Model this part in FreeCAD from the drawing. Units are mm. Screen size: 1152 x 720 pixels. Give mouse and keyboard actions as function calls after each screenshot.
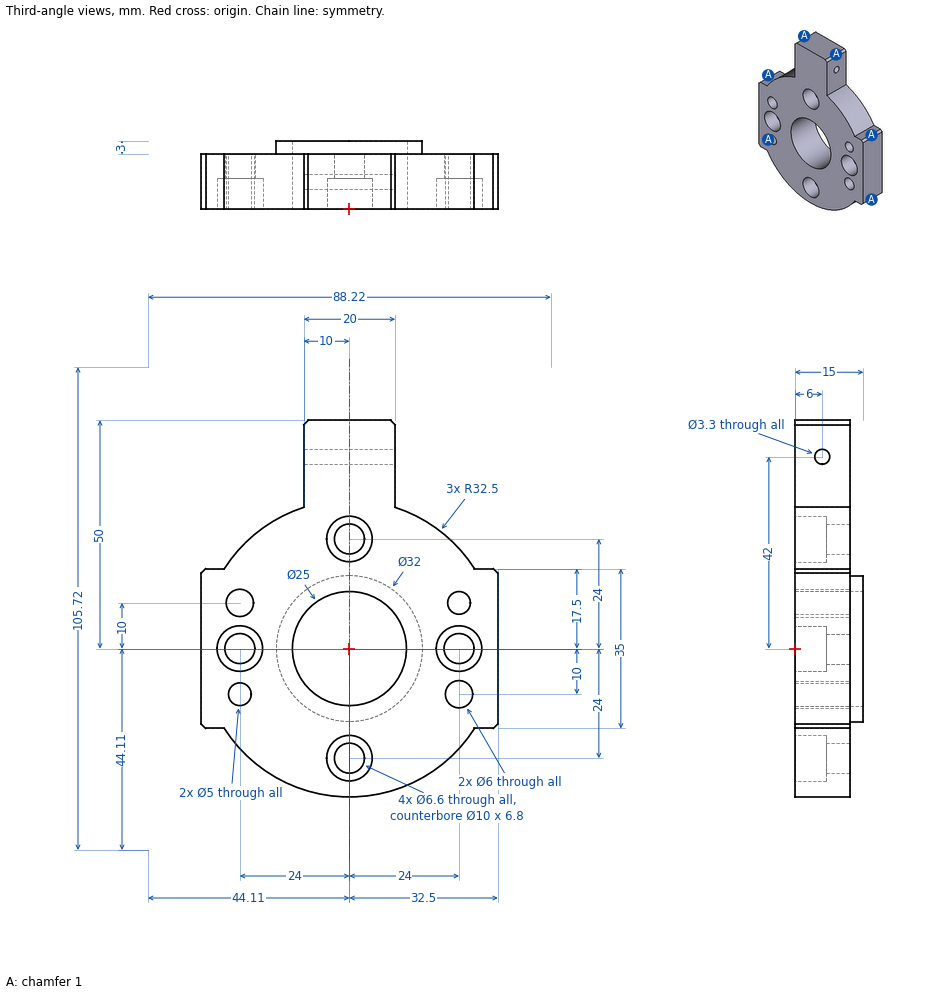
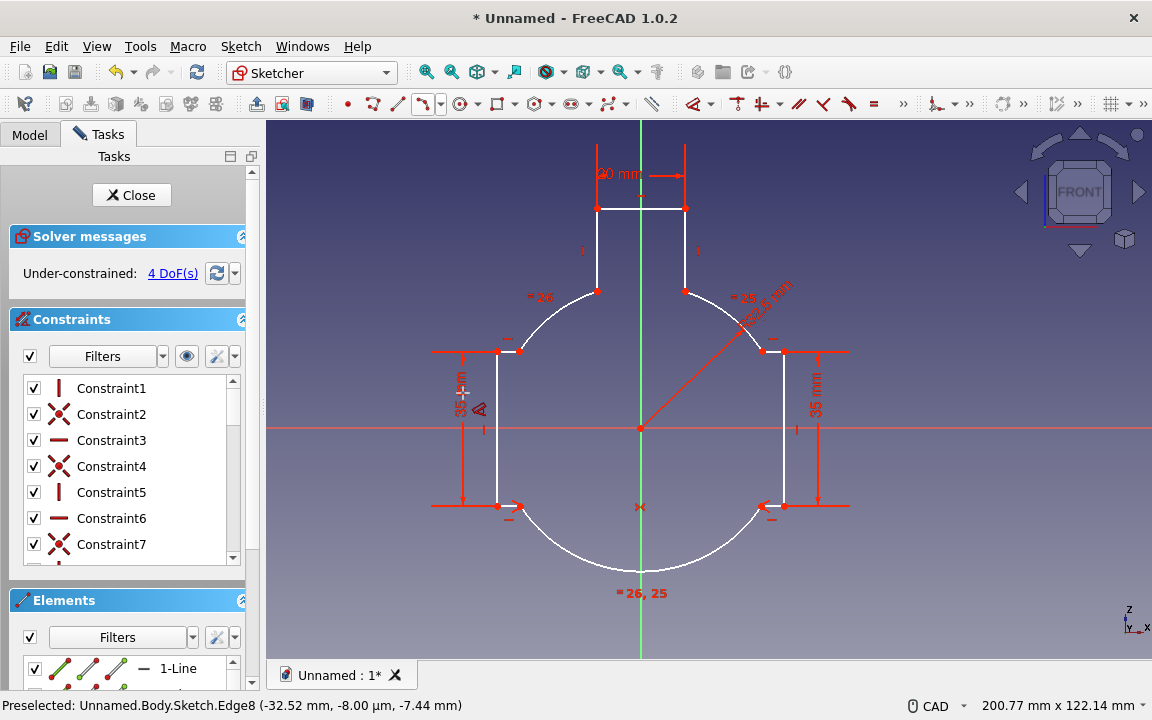
click(597, 292)
click(619, 258)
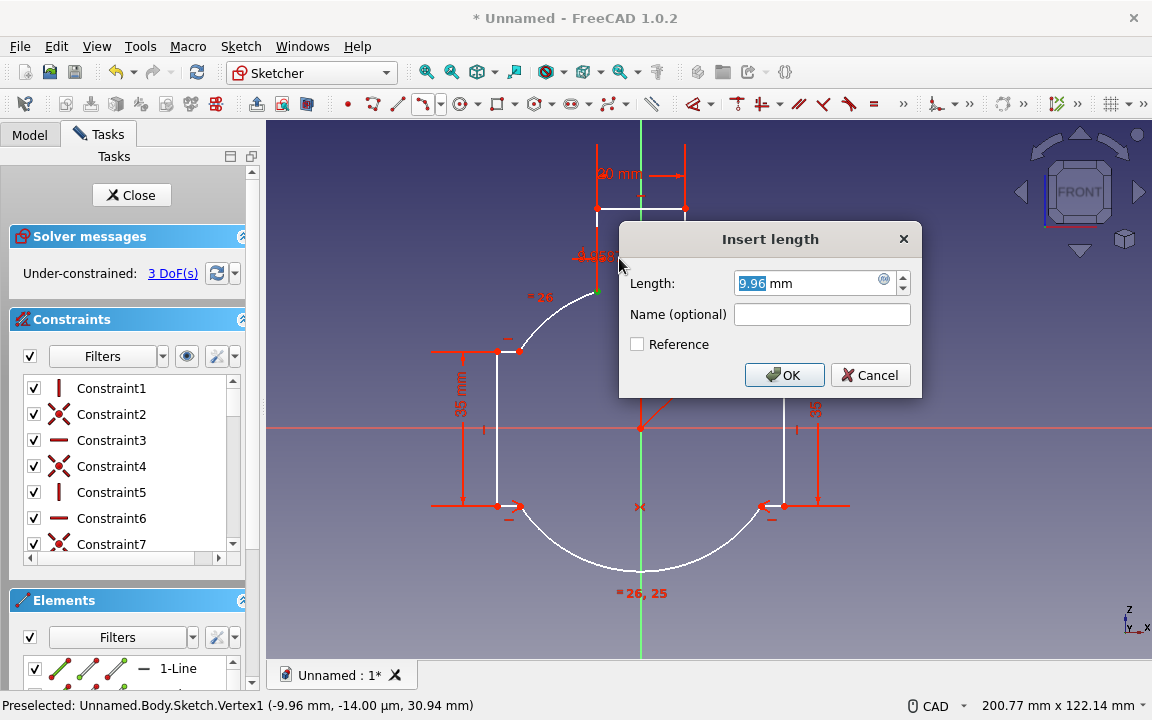
text(10)
key(Return)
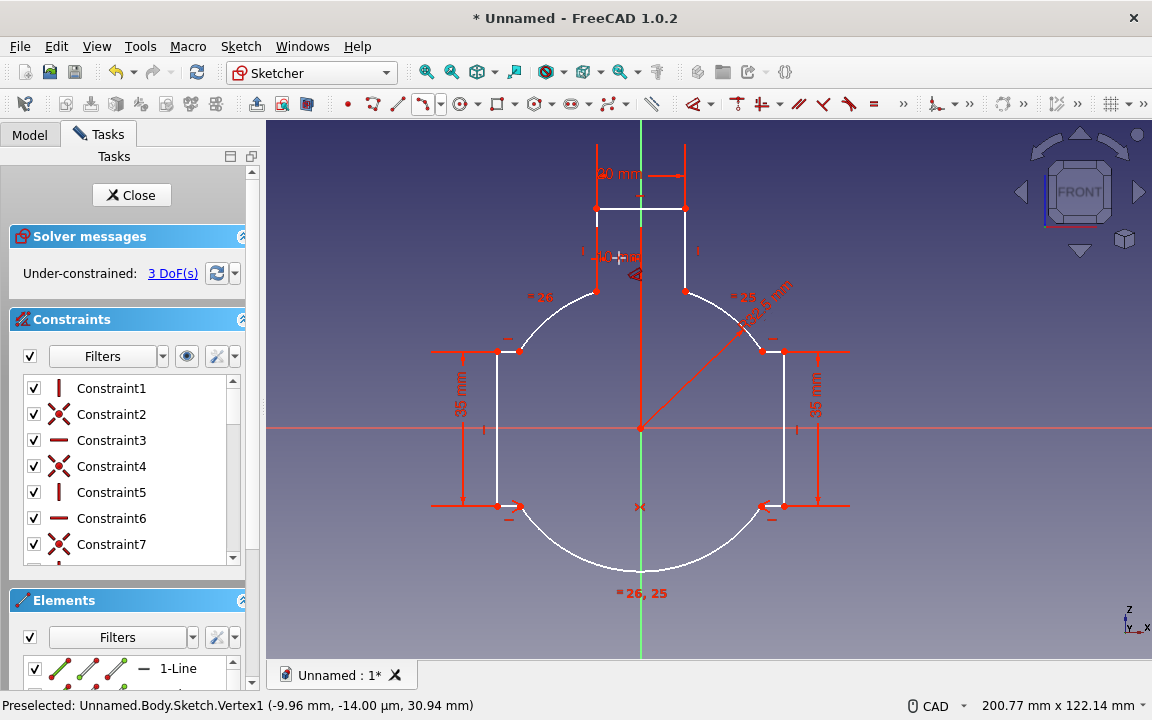
click(597, 209)
click(563, 369)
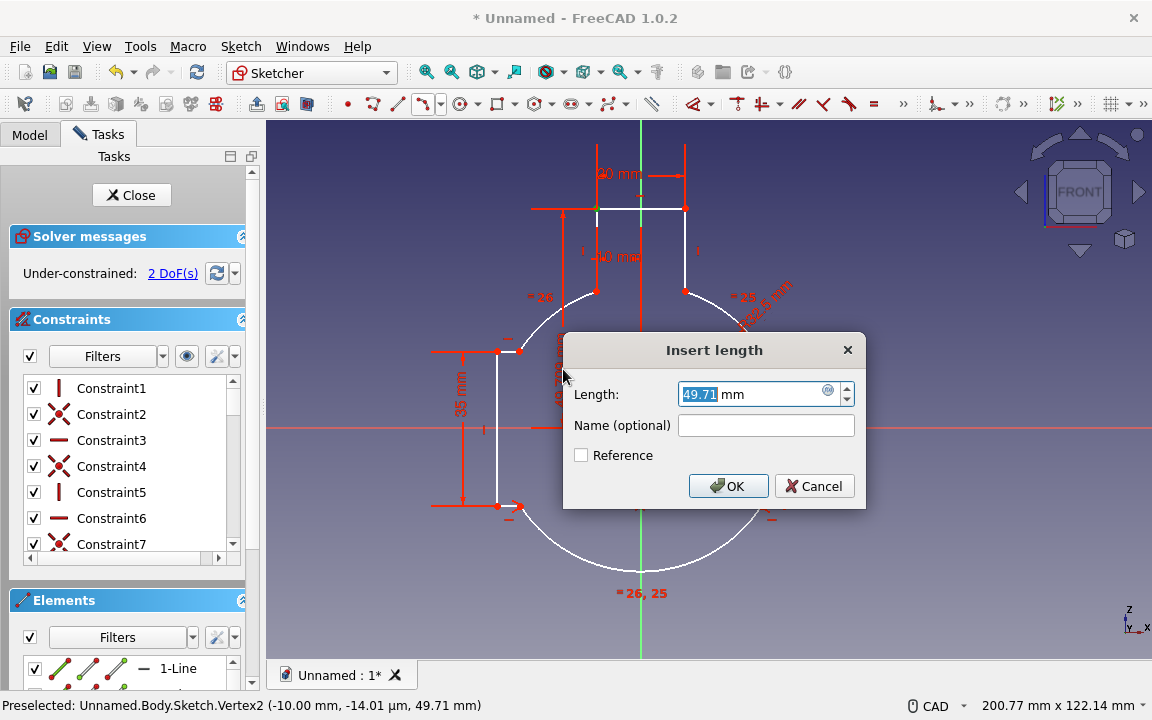
text(50)
key(Return)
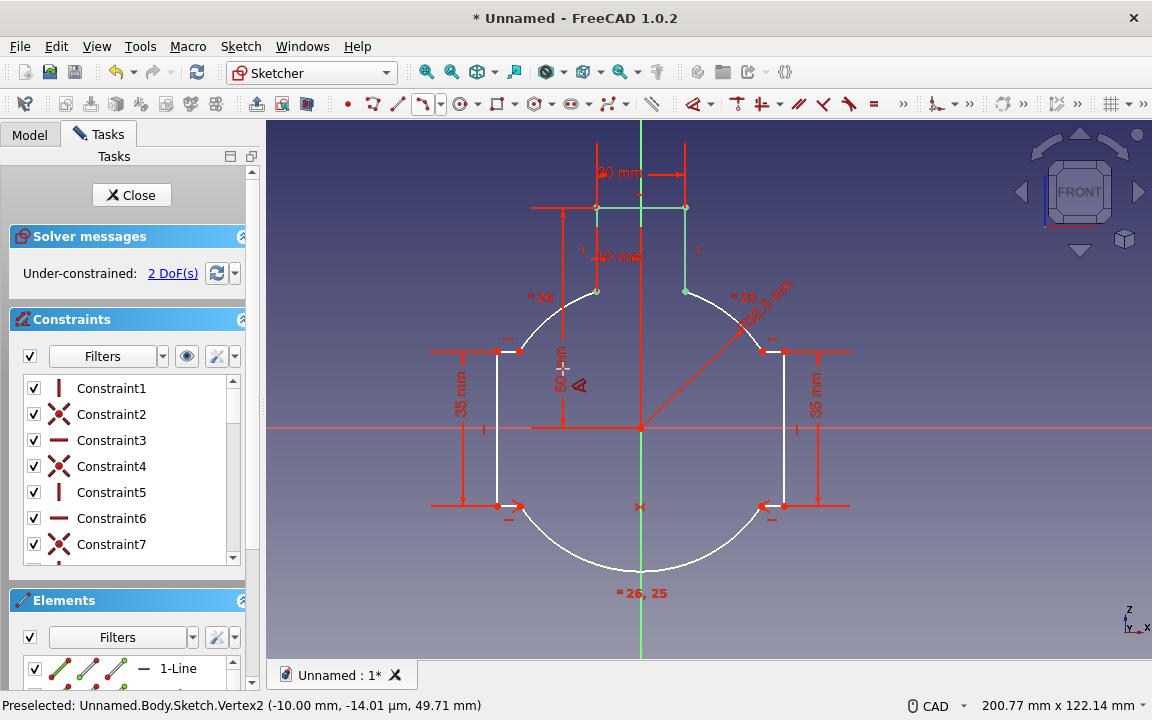
click(762, 352)
click(607, 390)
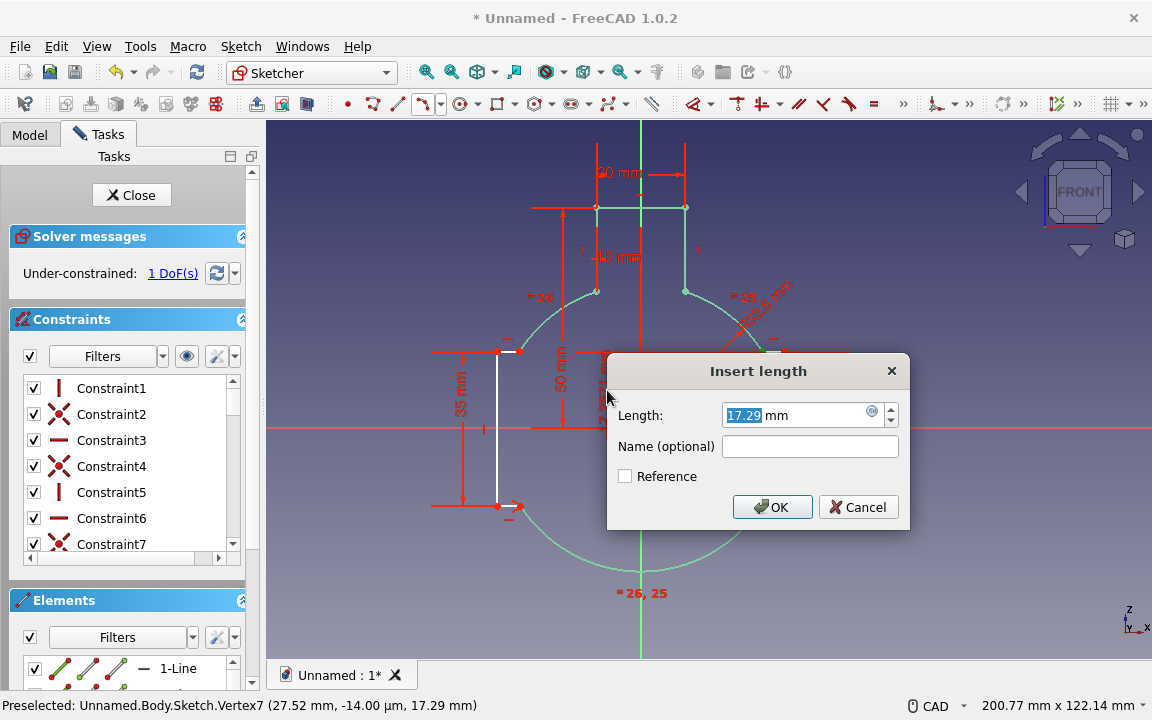
text(17.5)
key(Return)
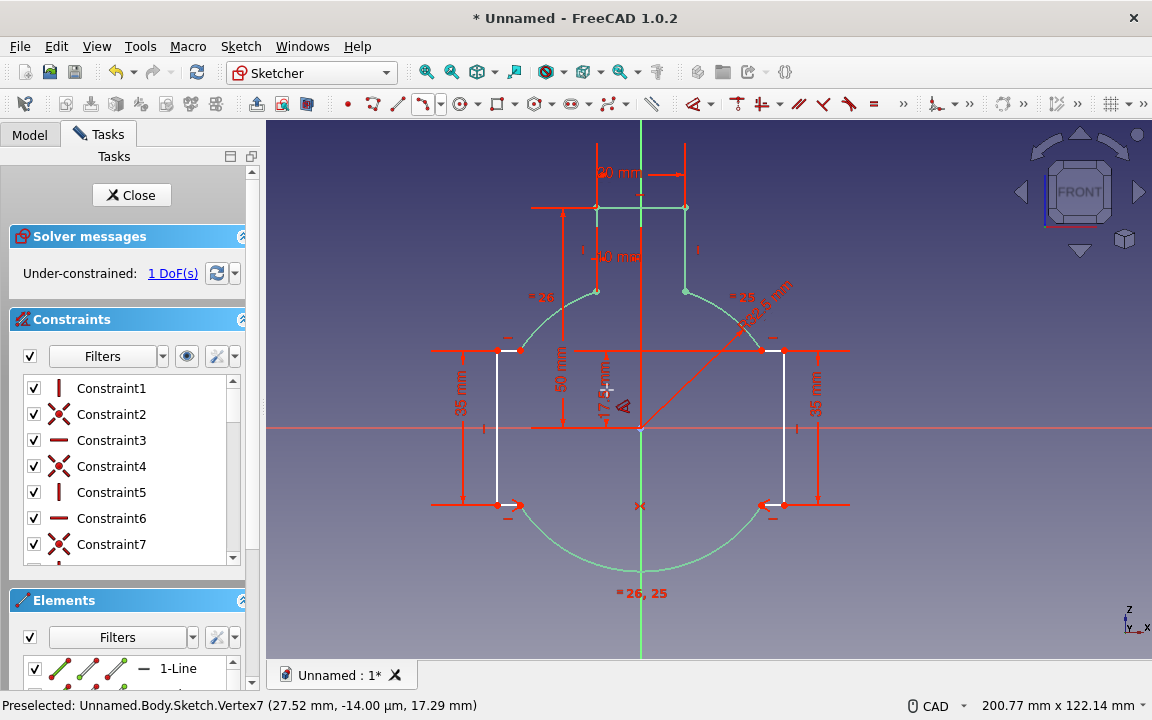
click(784, 351)
click(713, 462)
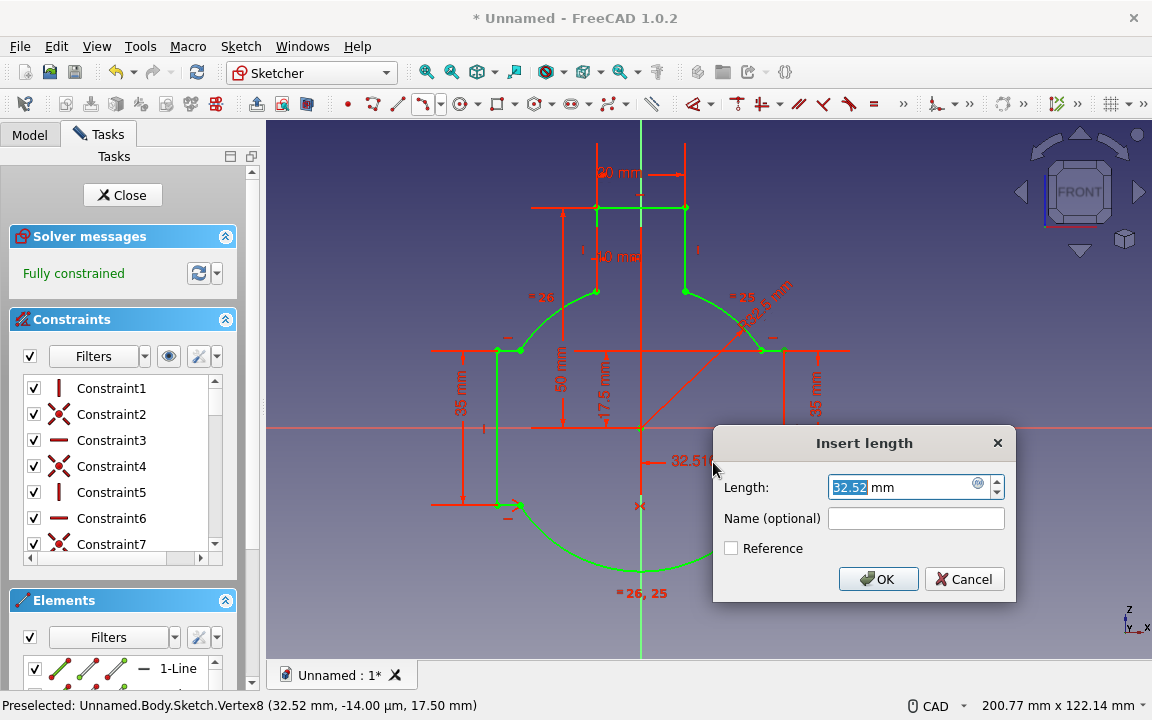
text(32.5)
key(Return)
key(Escape)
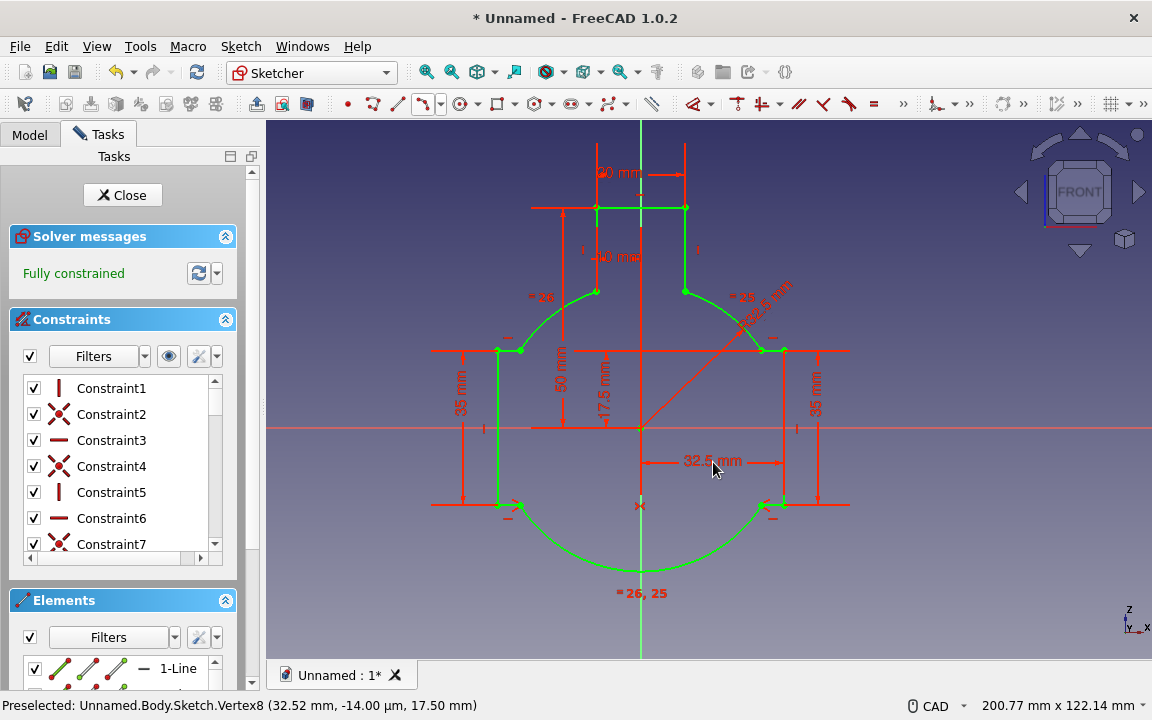
click(123, 195)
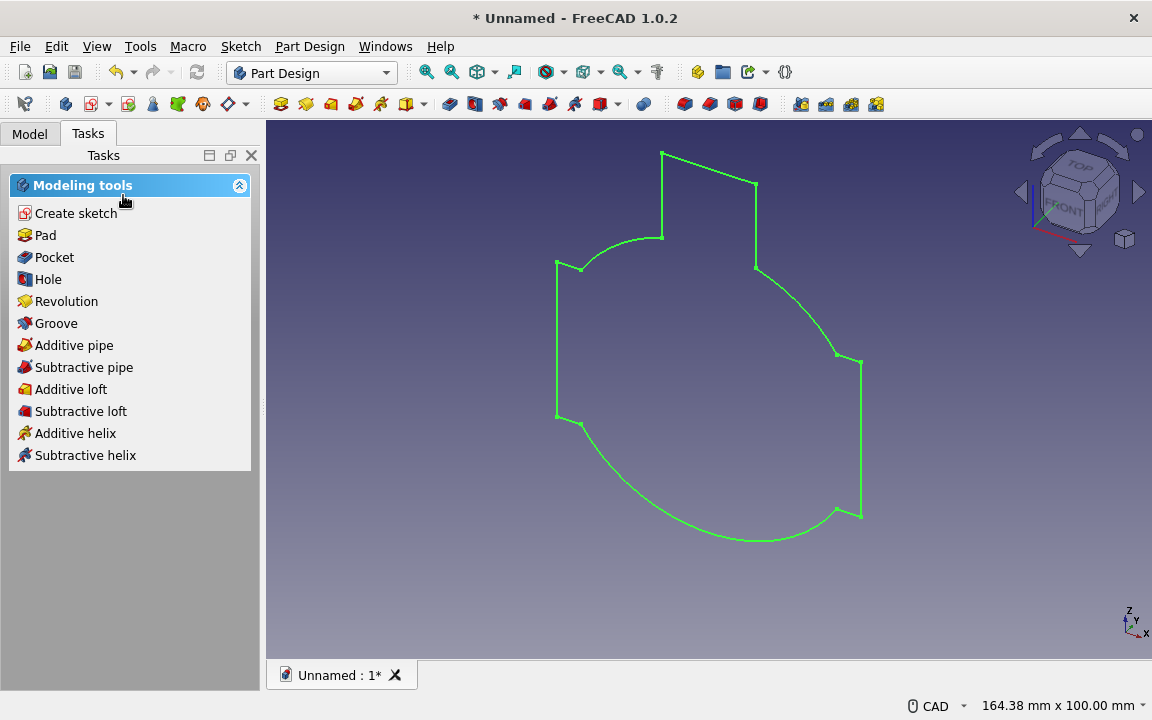
click(281, 104)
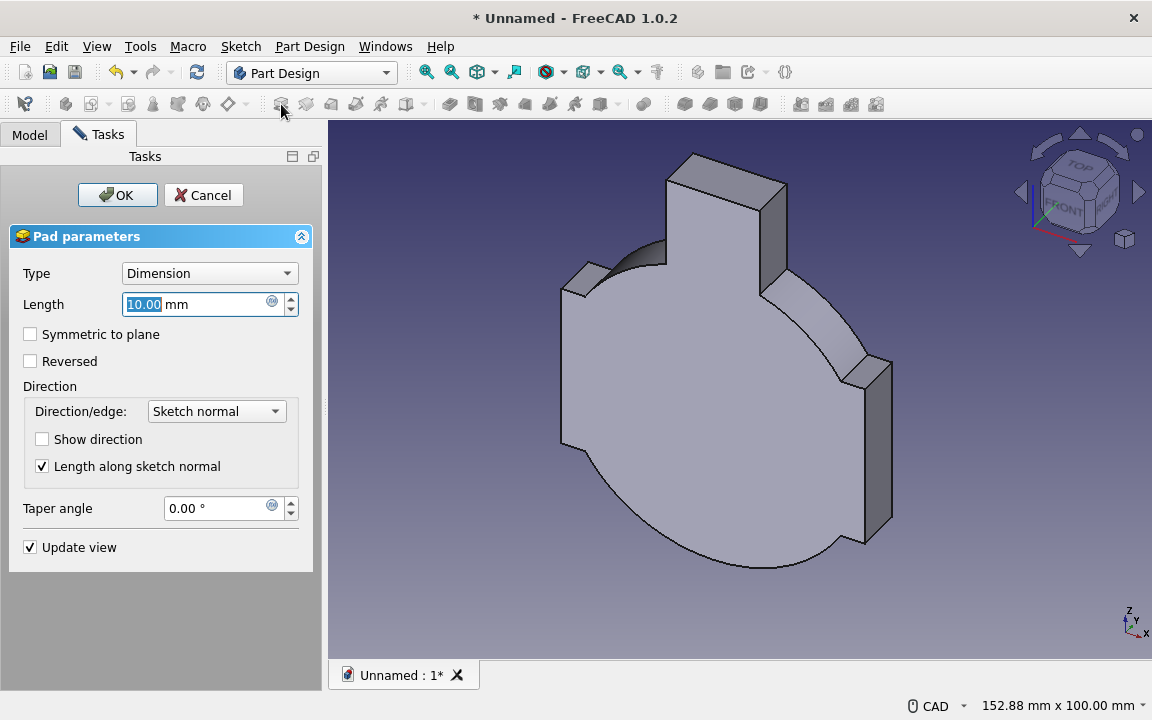
text(15)
key(Tab)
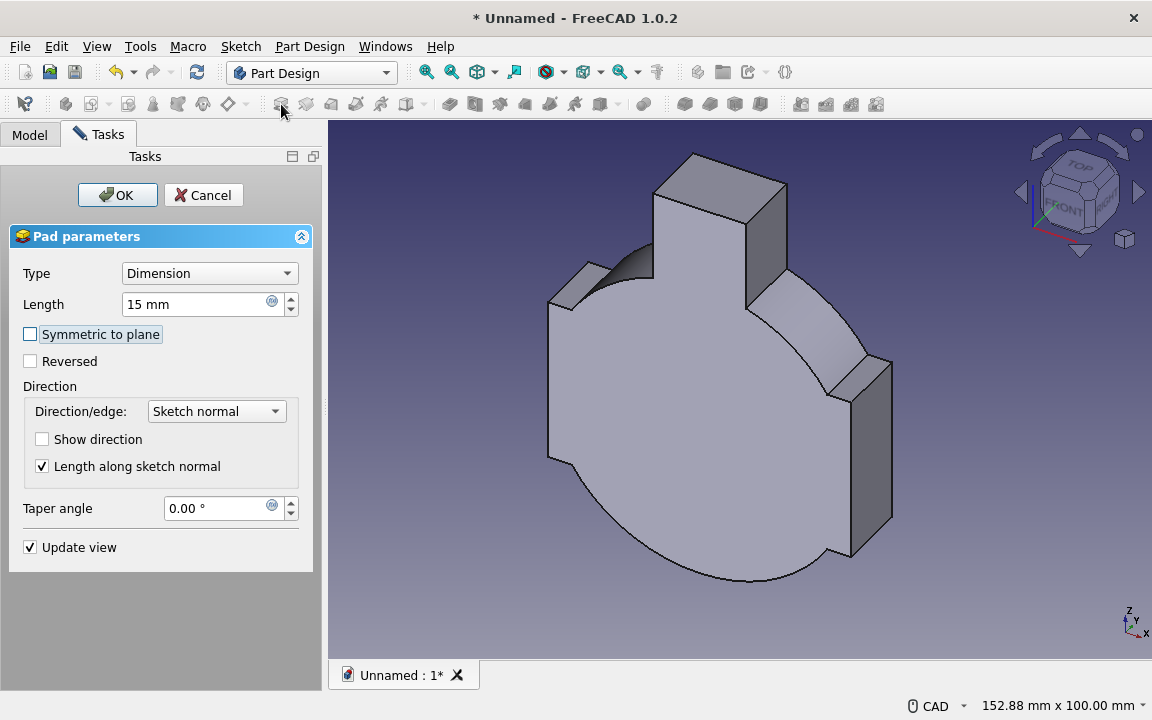
click(31, 361)